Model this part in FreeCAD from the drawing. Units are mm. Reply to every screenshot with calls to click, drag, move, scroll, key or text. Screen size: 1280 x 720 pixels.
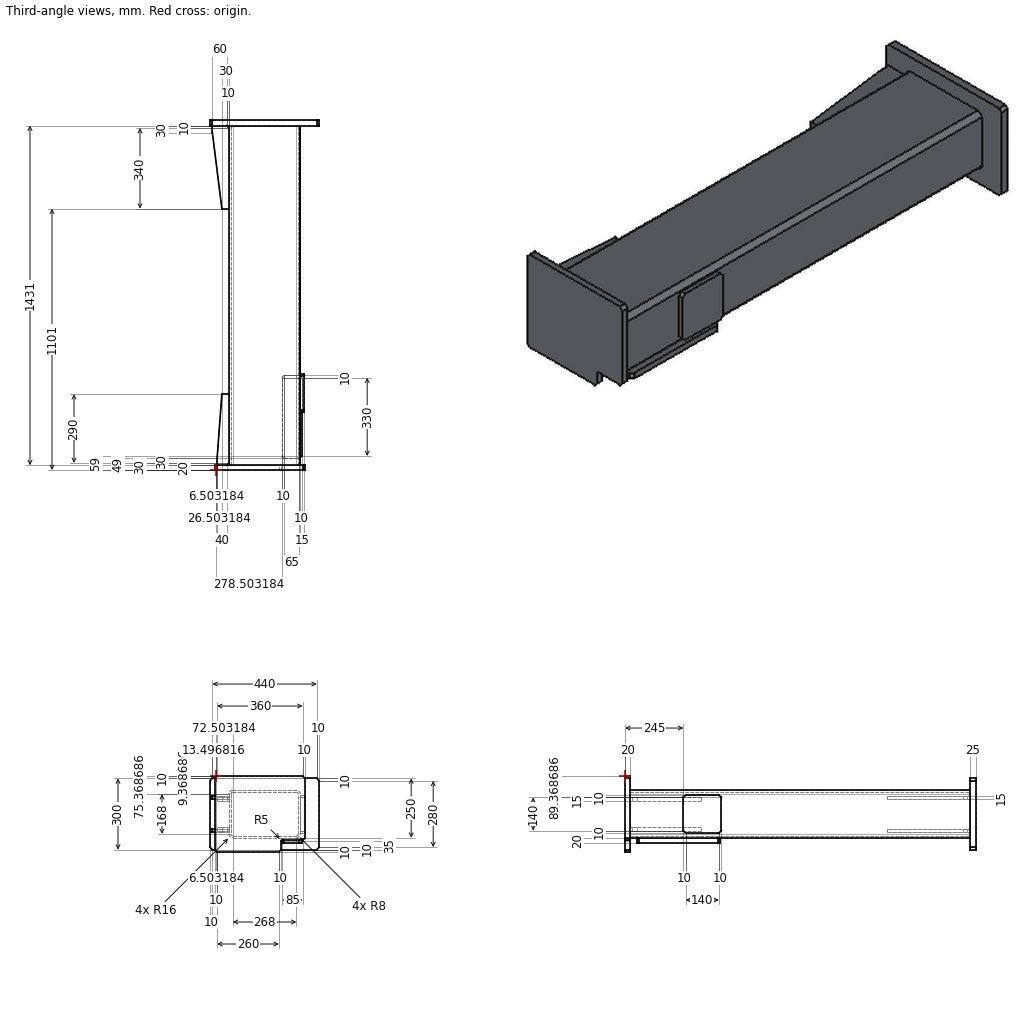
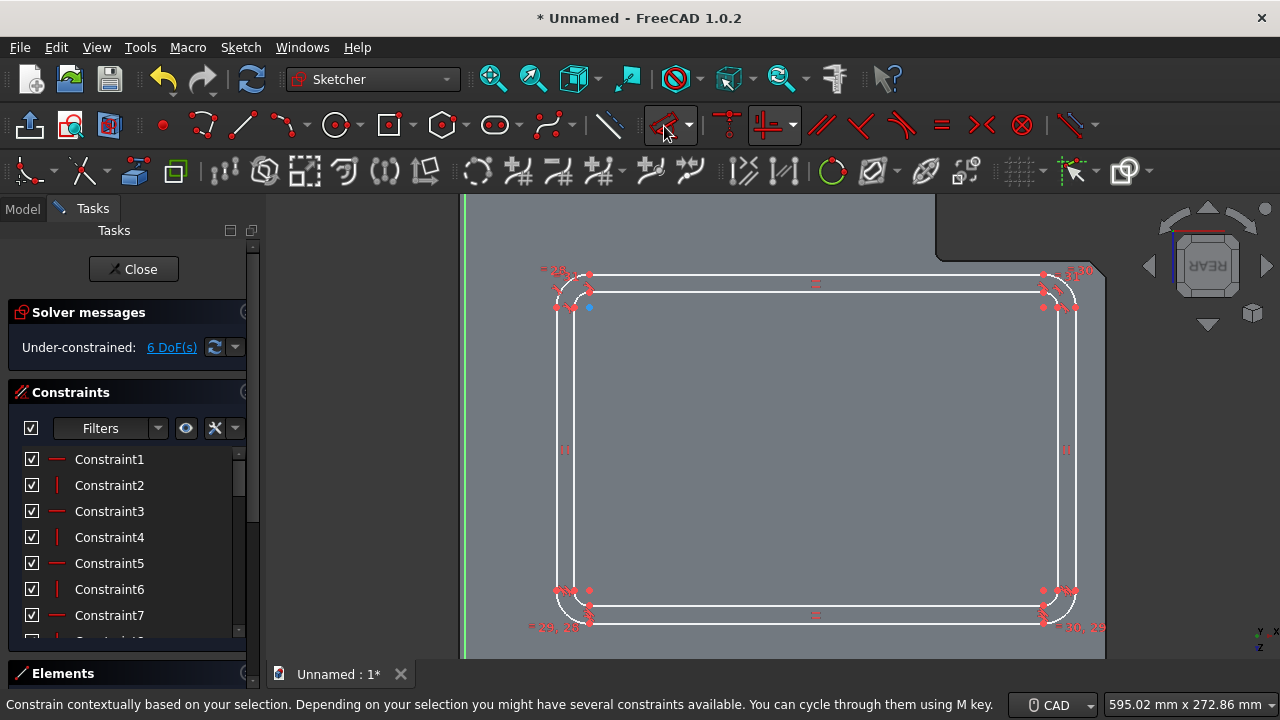
scroll(574, 278, up, 2)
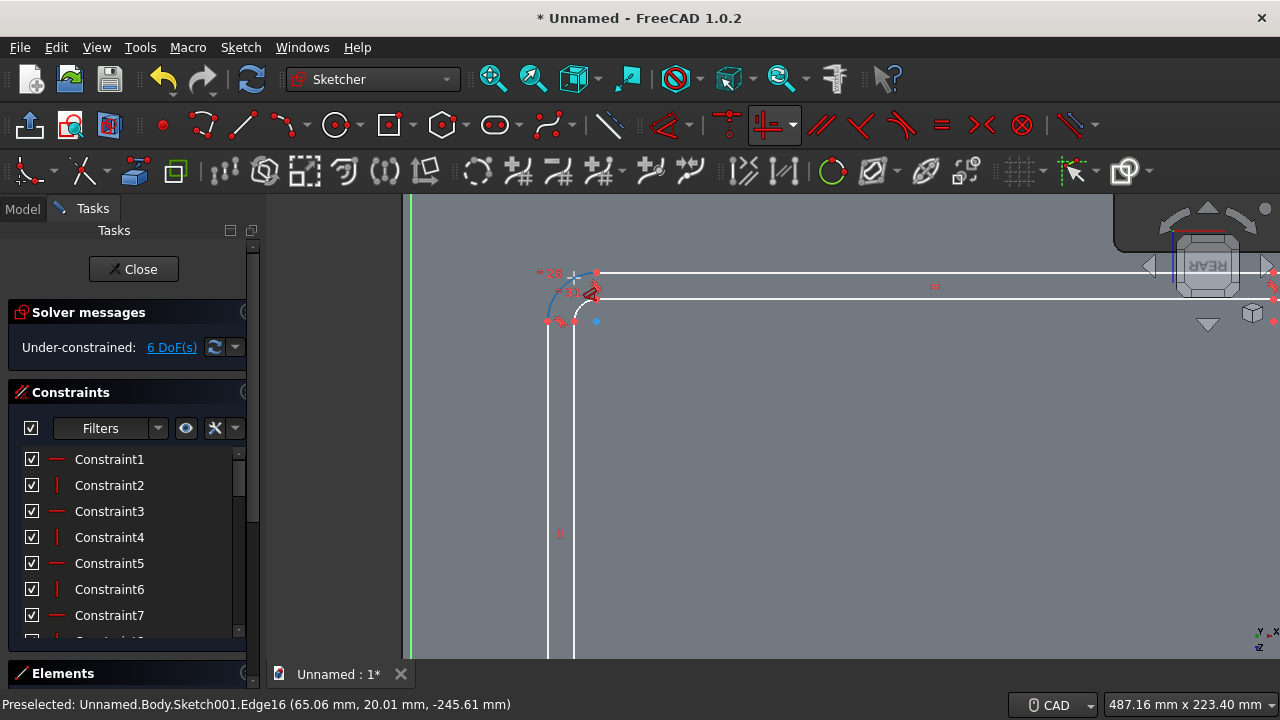
click(574, 278)
click(559, 250)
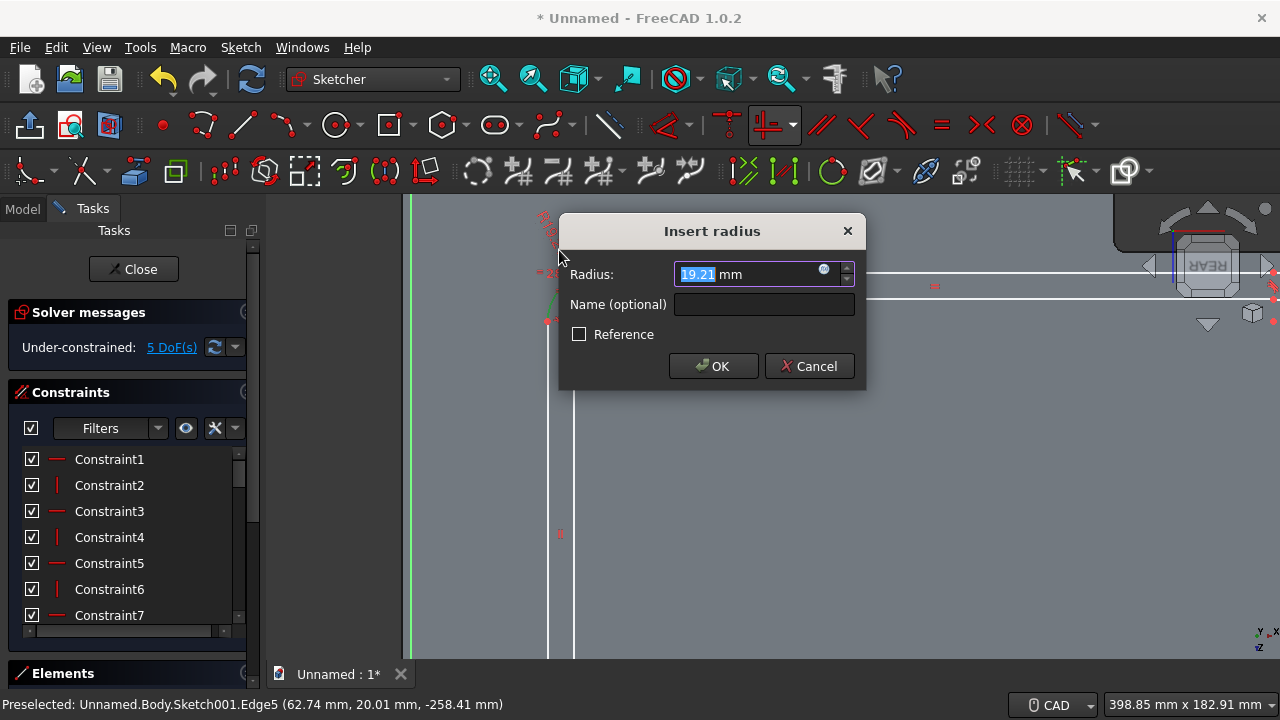
text(16)
key(Return)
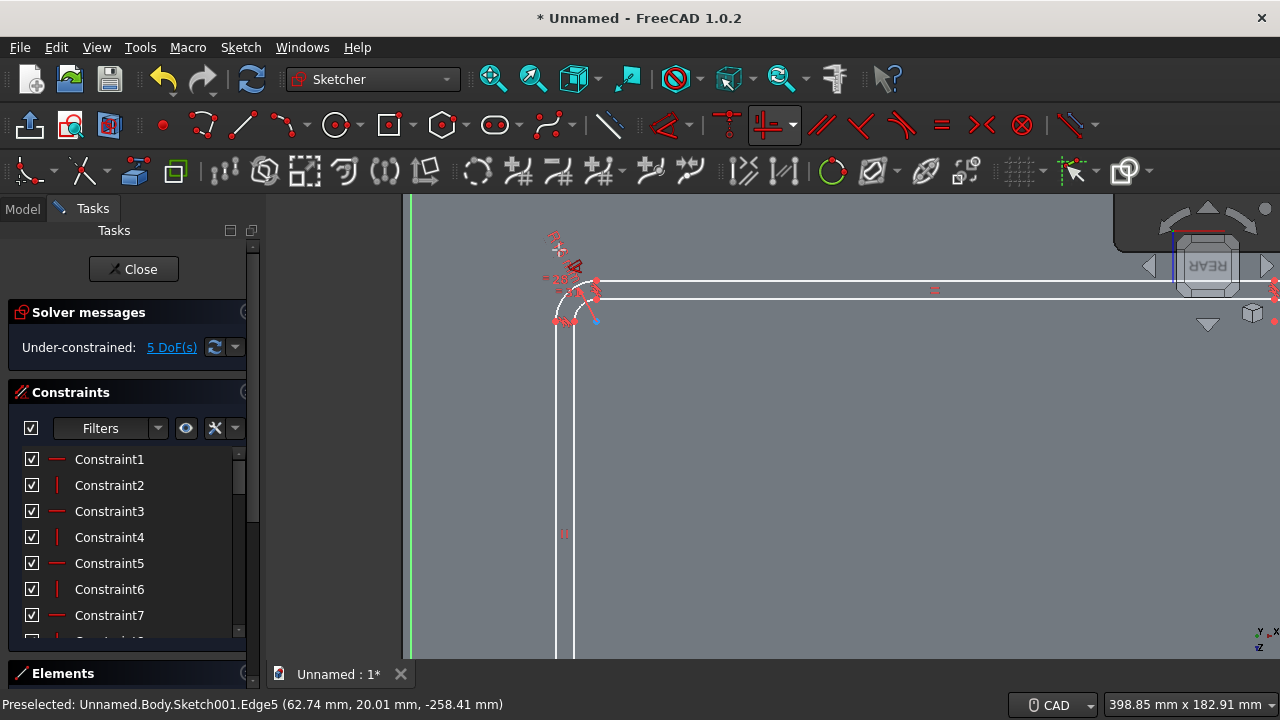
scroll(574, 279, down, 4)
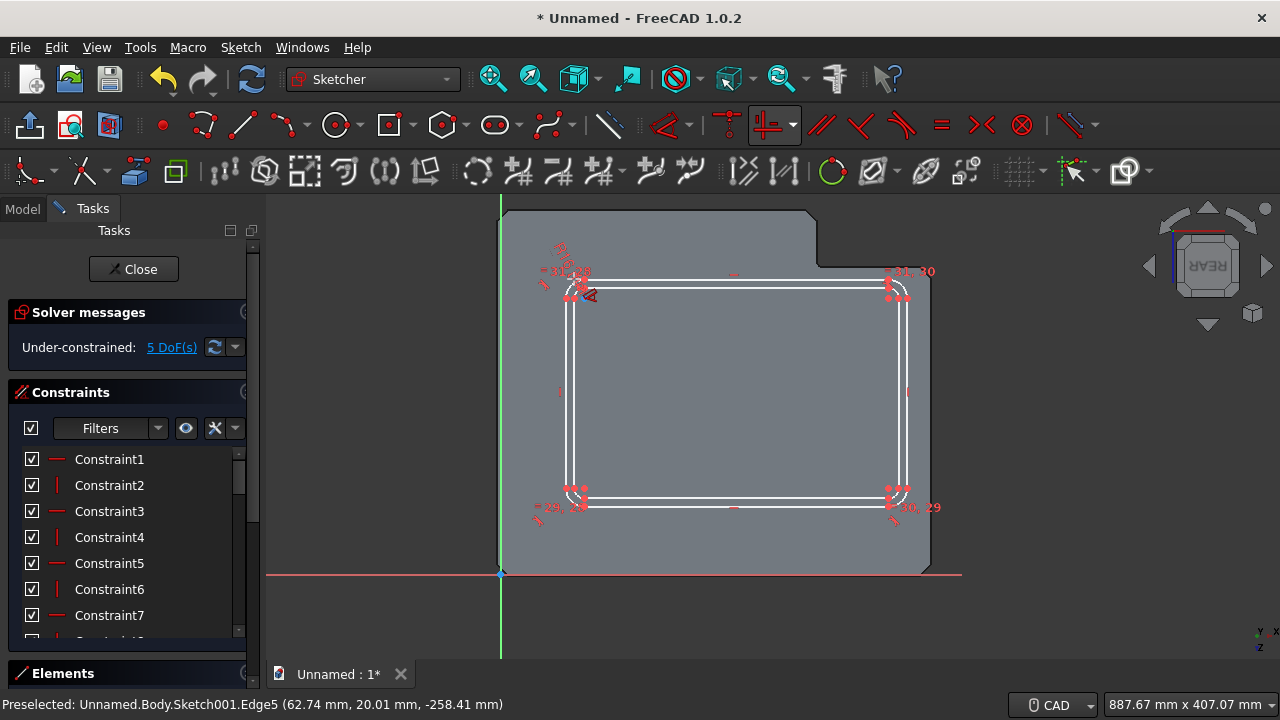
scroll(898, 294, up, 8)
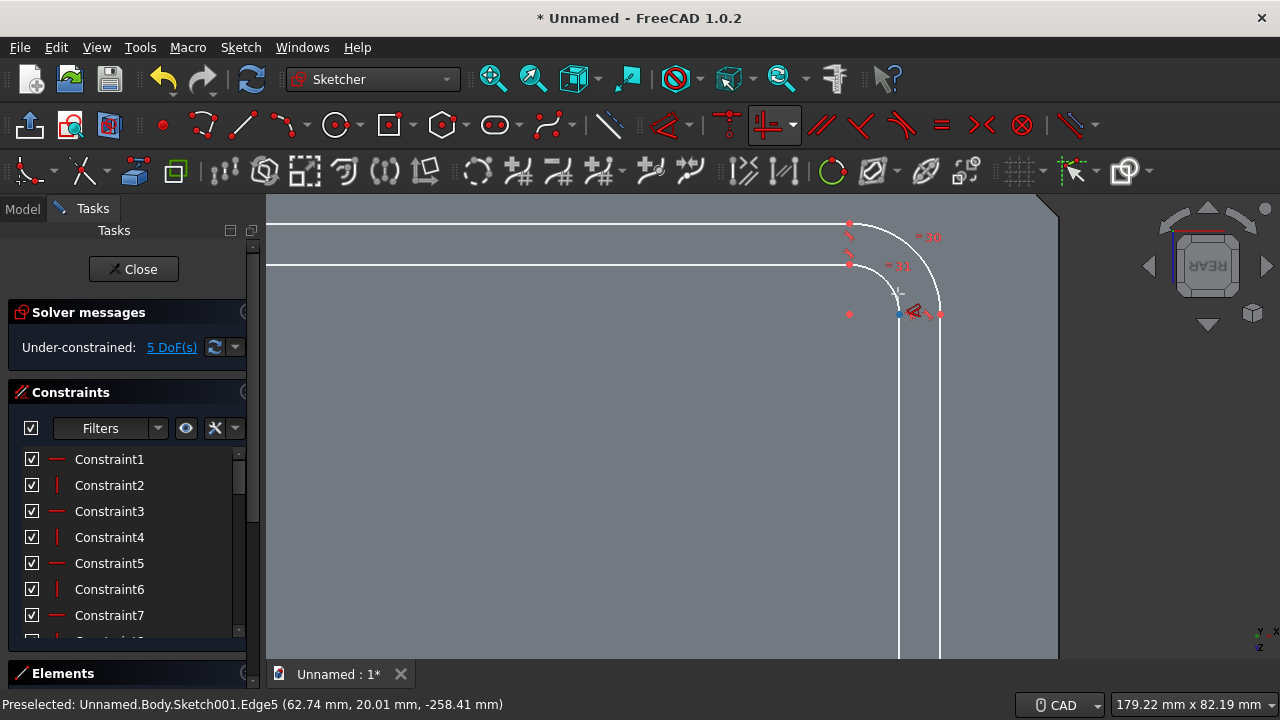
click(894, 292)
click(920, 356)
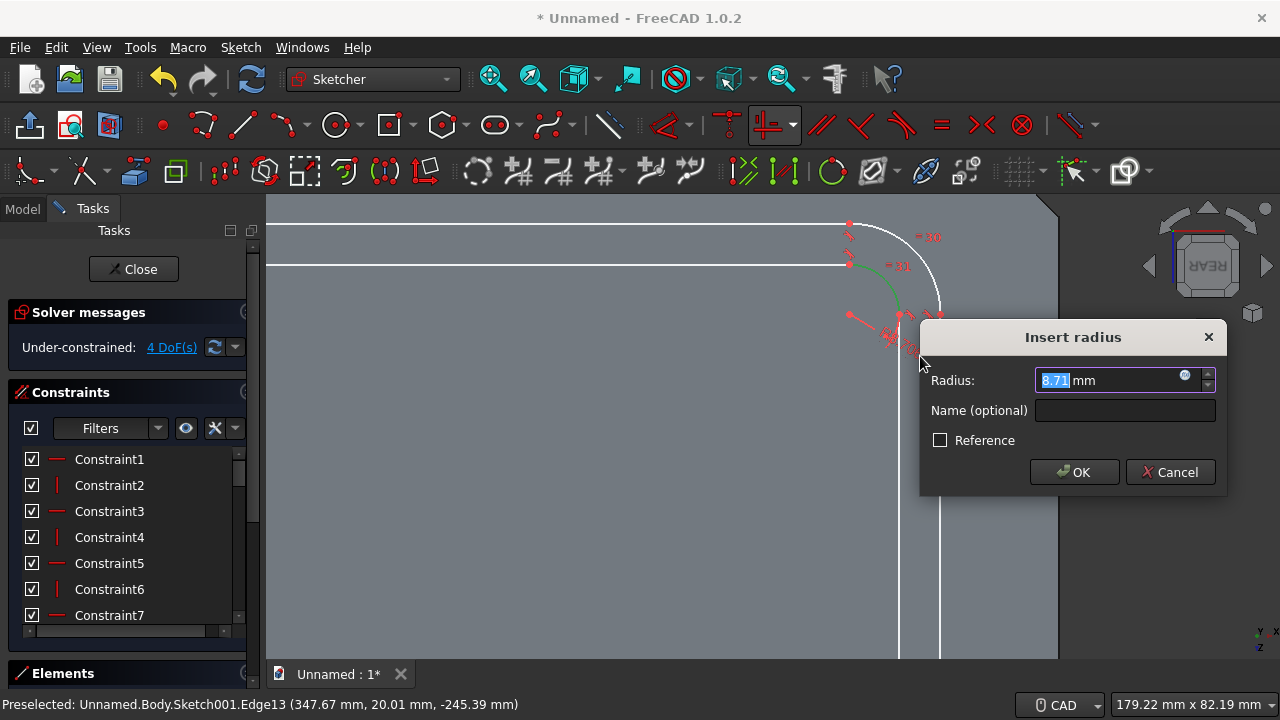
text(8)
key(Return)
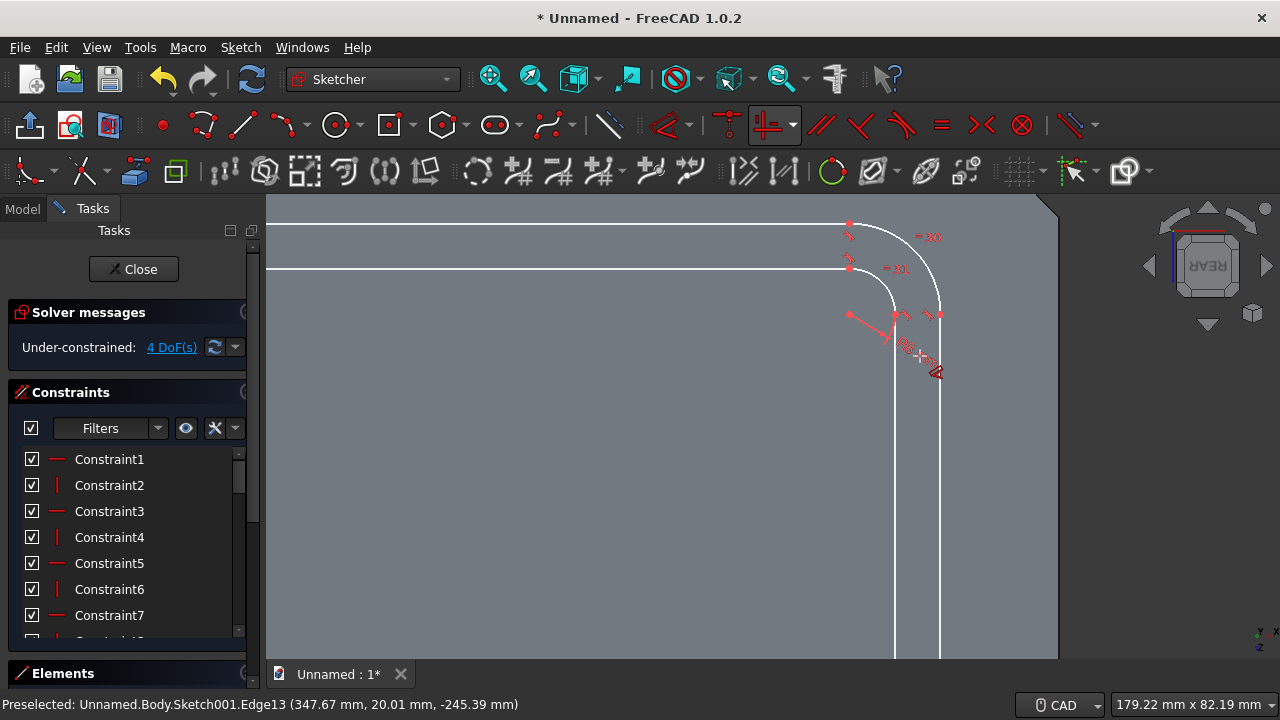
scroll(899, 294, down, 8)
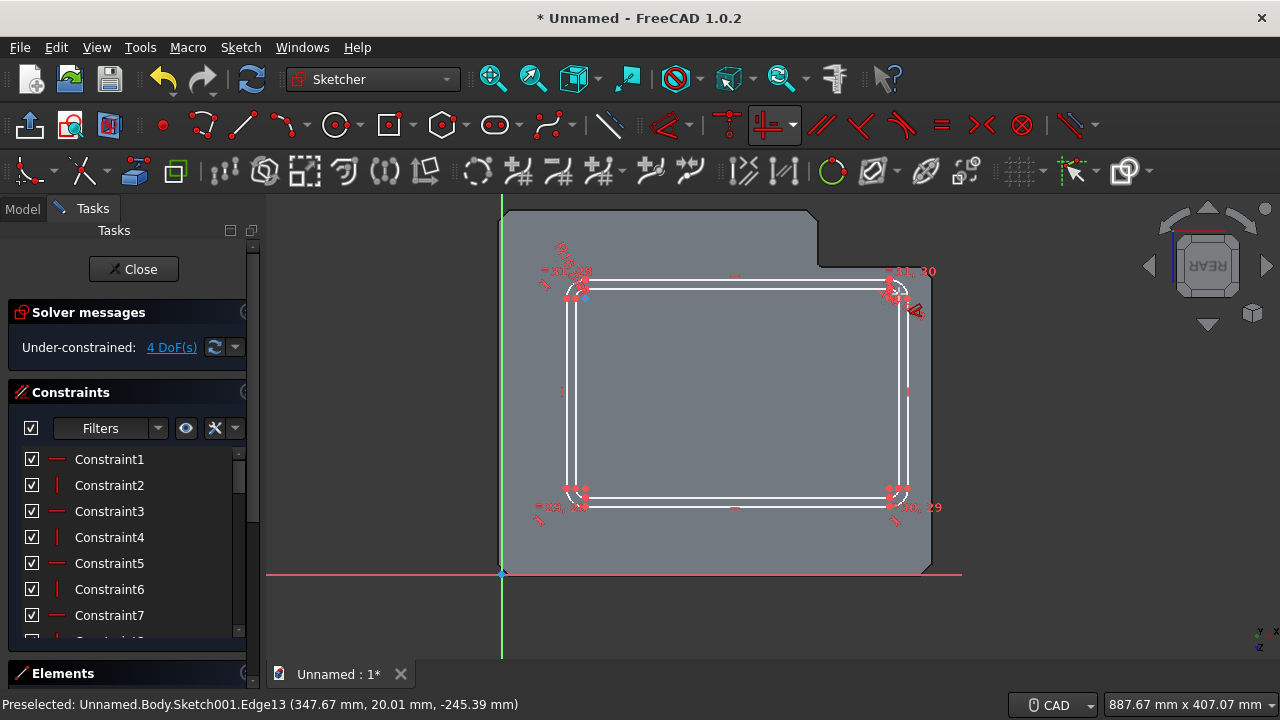
scroll(798, 280, up, 3)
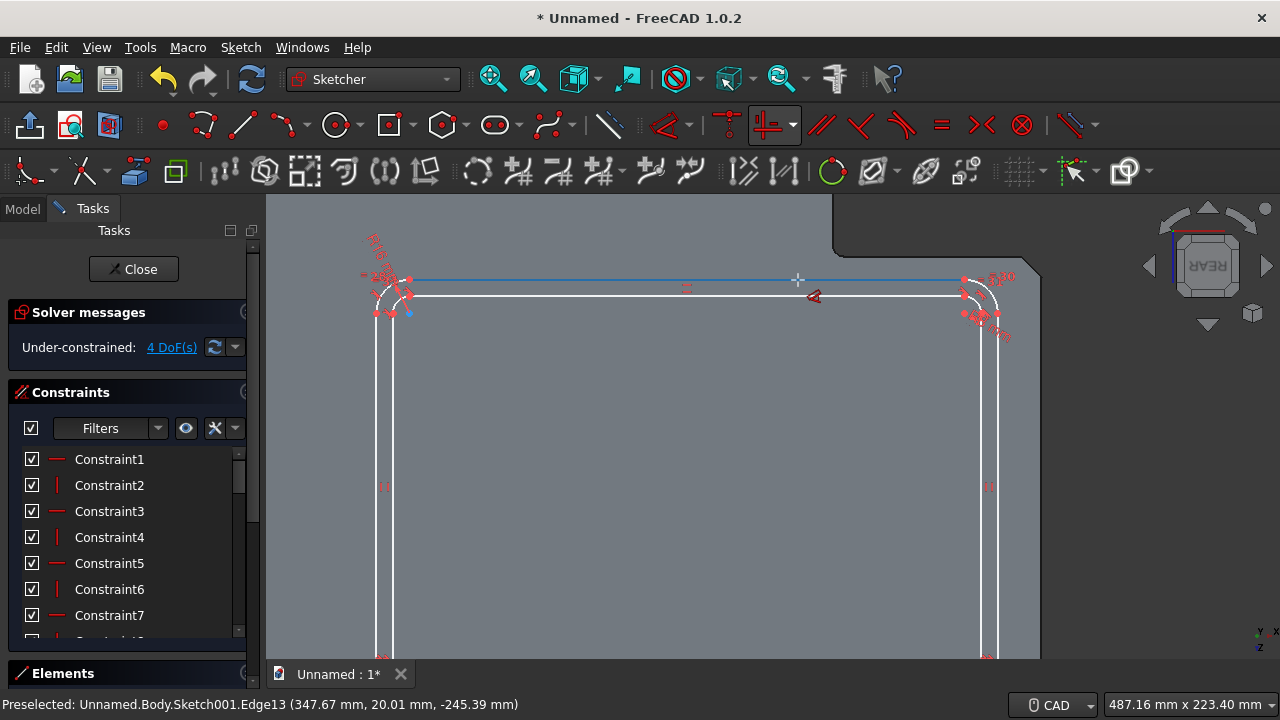
click(798, 280)
click(687, 246)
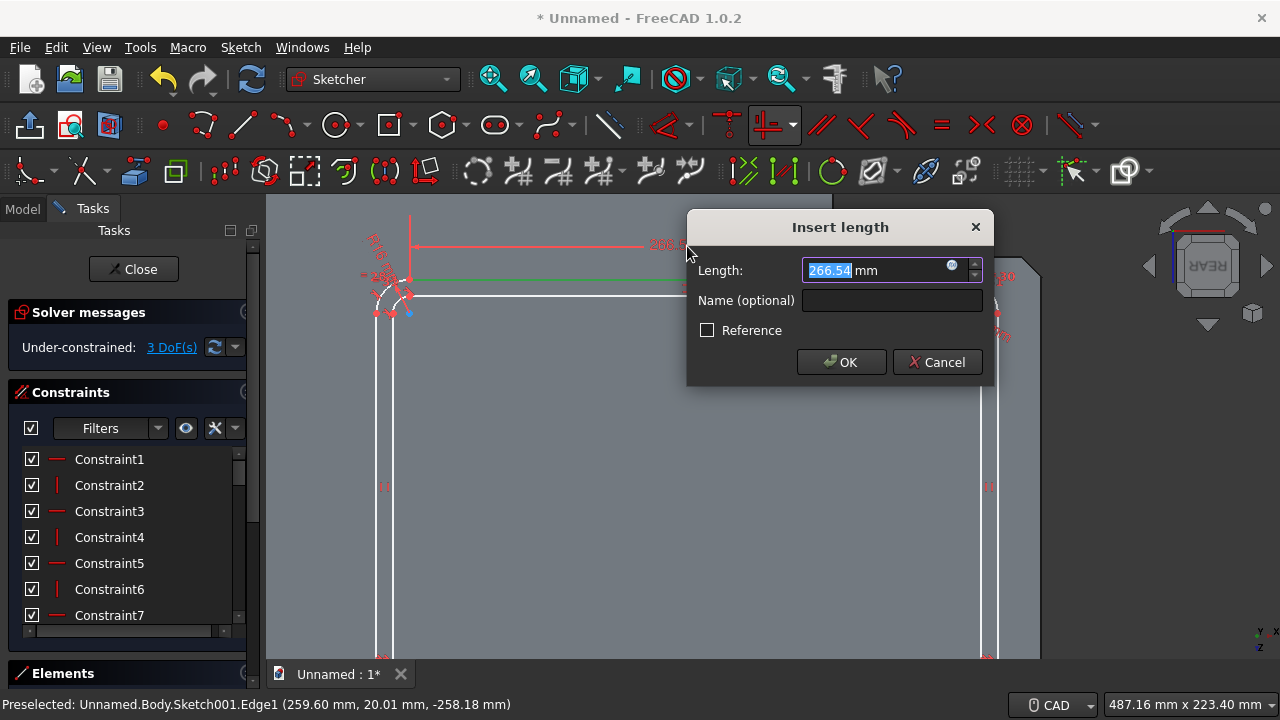
text(268)
key(Return)